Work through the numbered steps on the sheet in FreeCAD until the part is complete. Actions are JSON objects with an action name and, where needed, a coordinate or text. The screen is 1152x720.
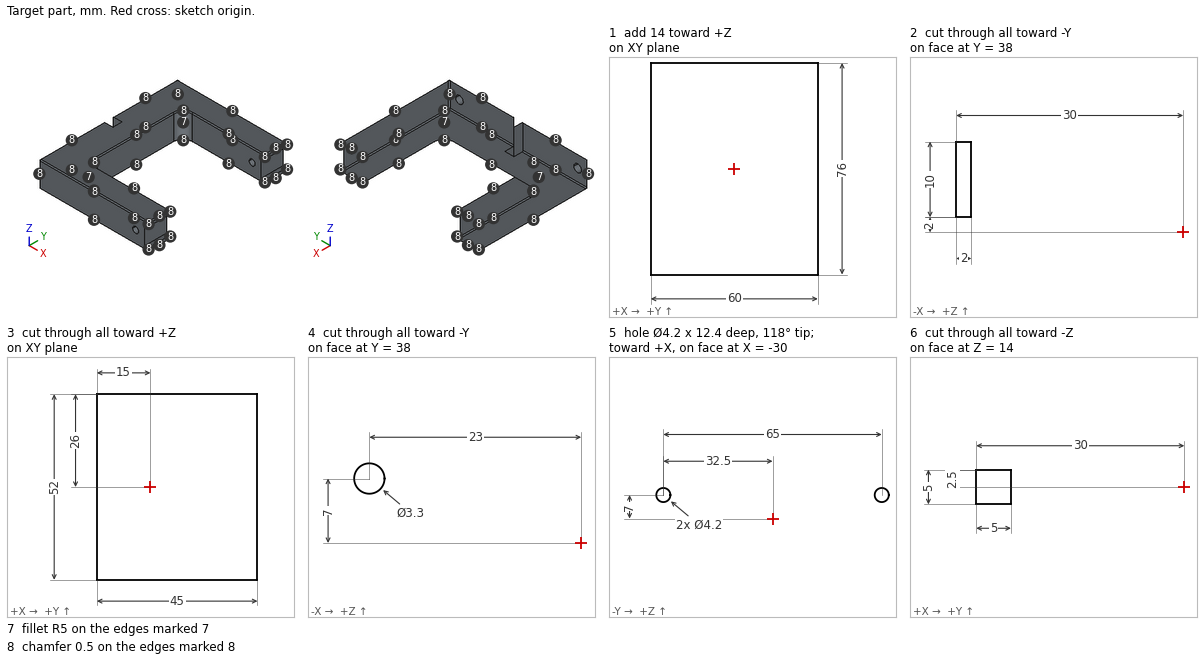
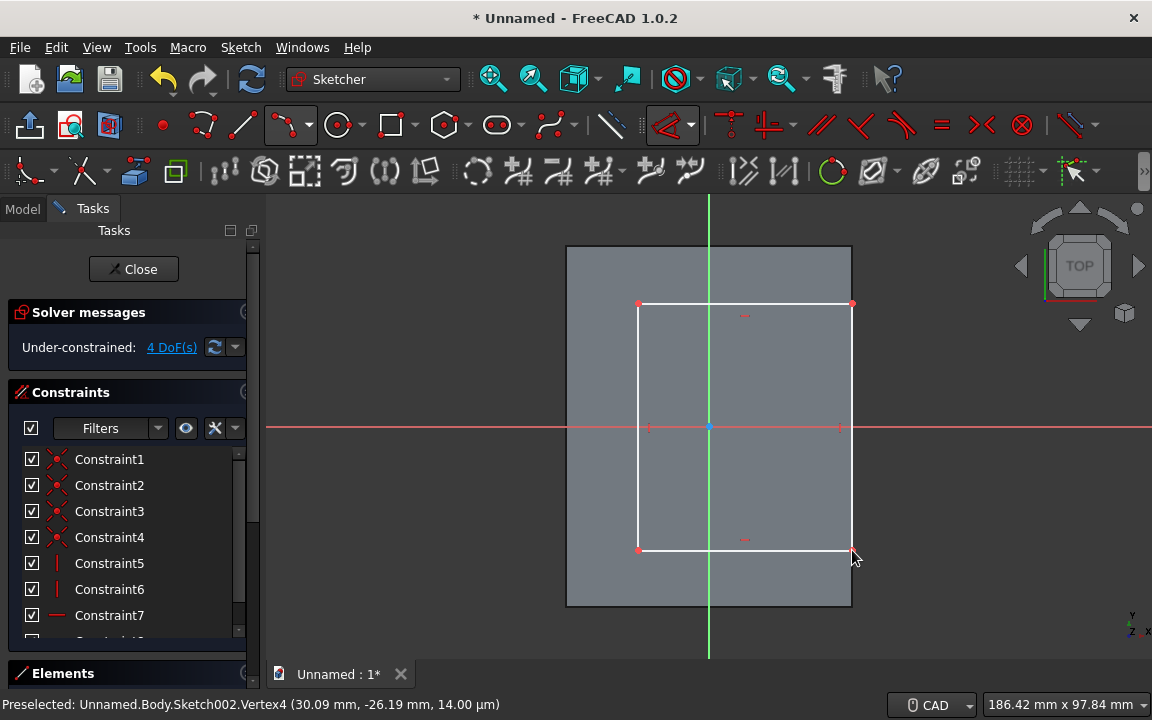
{"action": "left_click", "coordinate": [638, 378]}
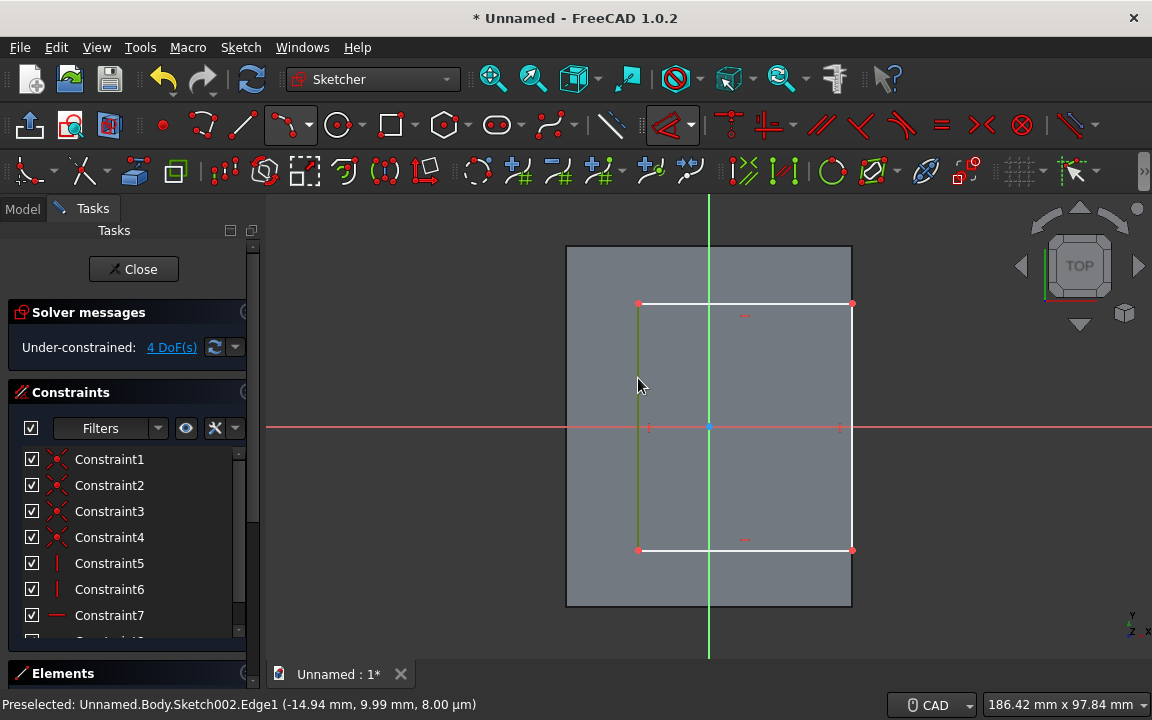
{"action": "key", "text": "i"}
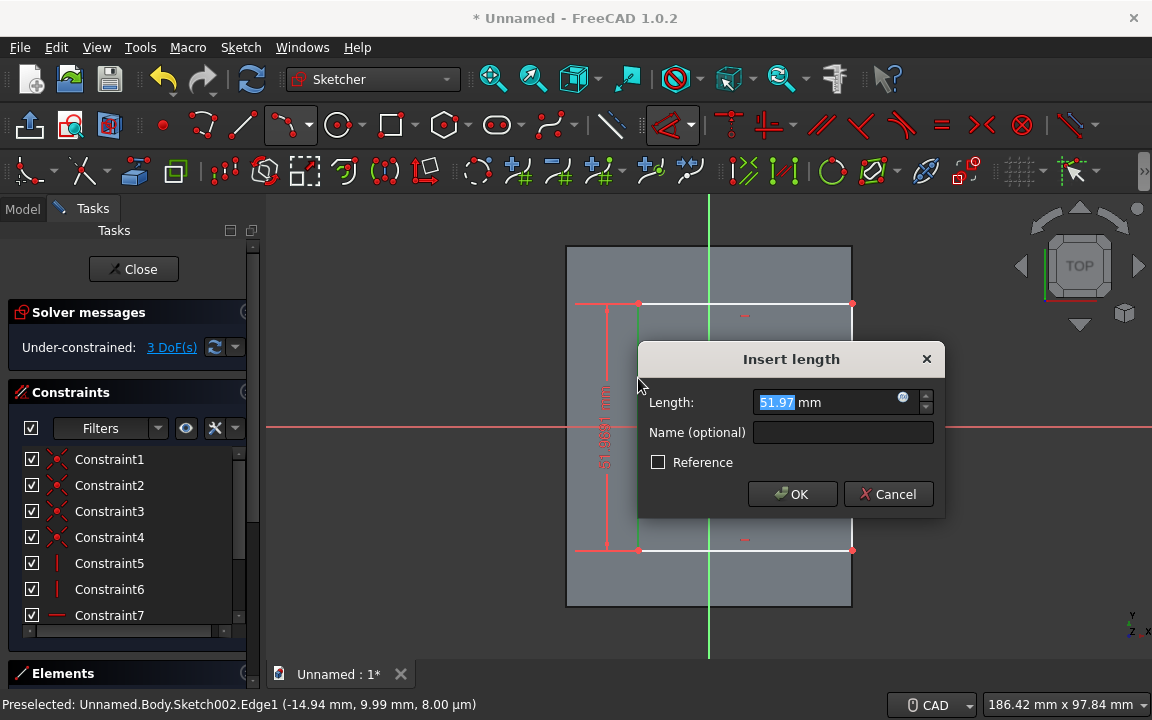
{"action": "type", "text": "52"}
{"action": "key", "text": "Return"}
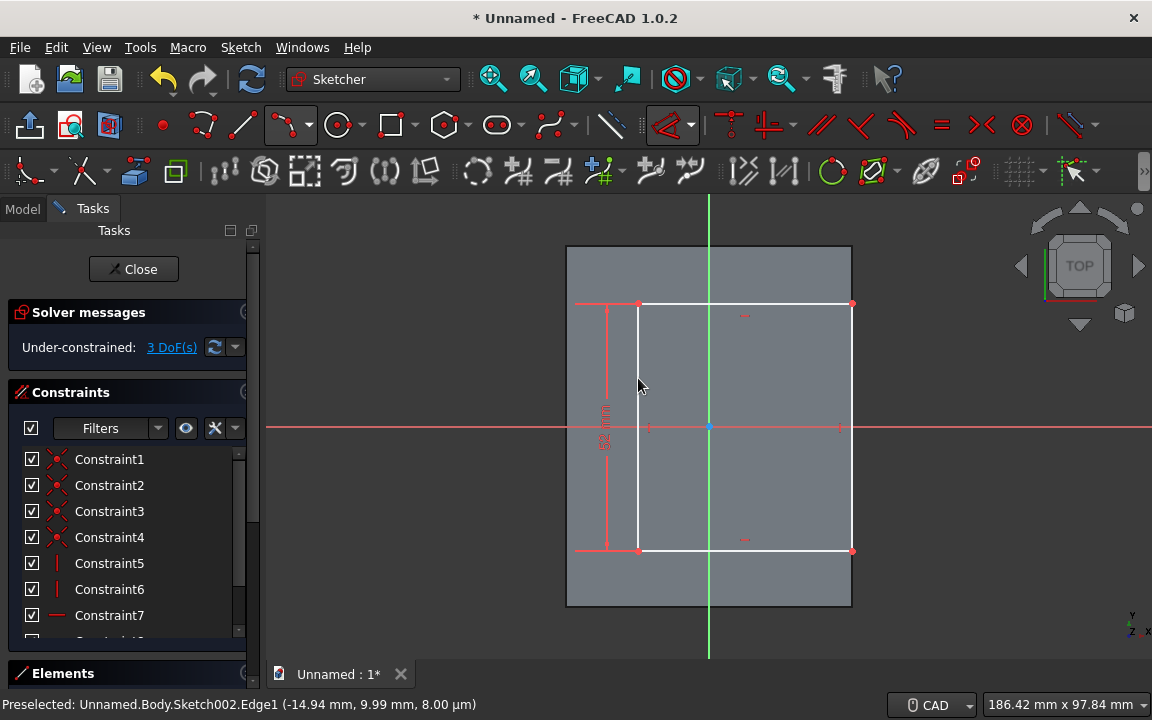
{"action": "left_click", "coordinate": [788, 551]}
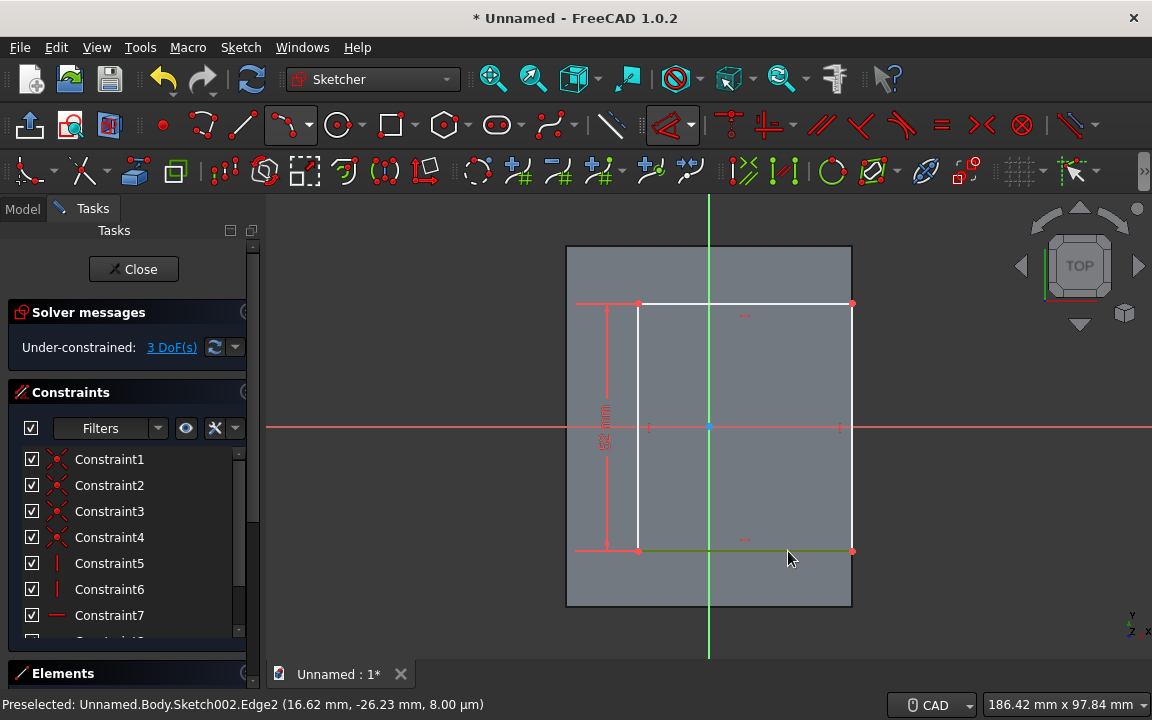
{"action": "key", "text": "l"}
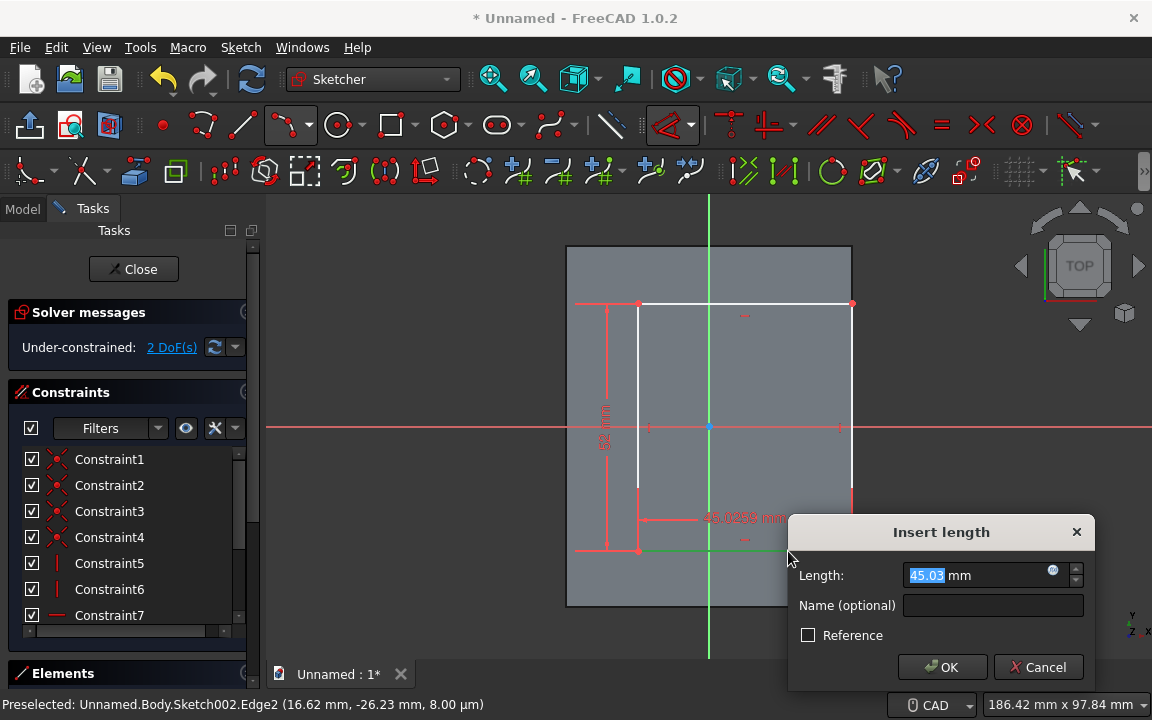
{"action": "type", "text": "45"}
{"action": "key", "text": "Return"}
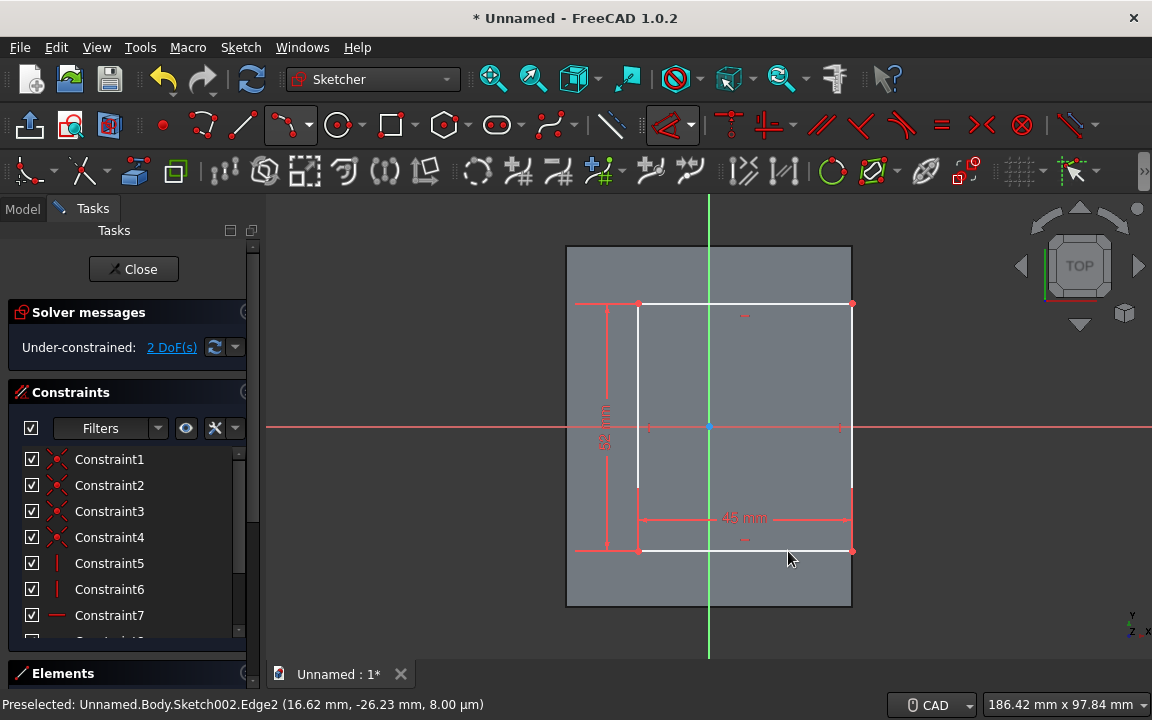
{"action": "left_click", "coordinate": [638, 304]}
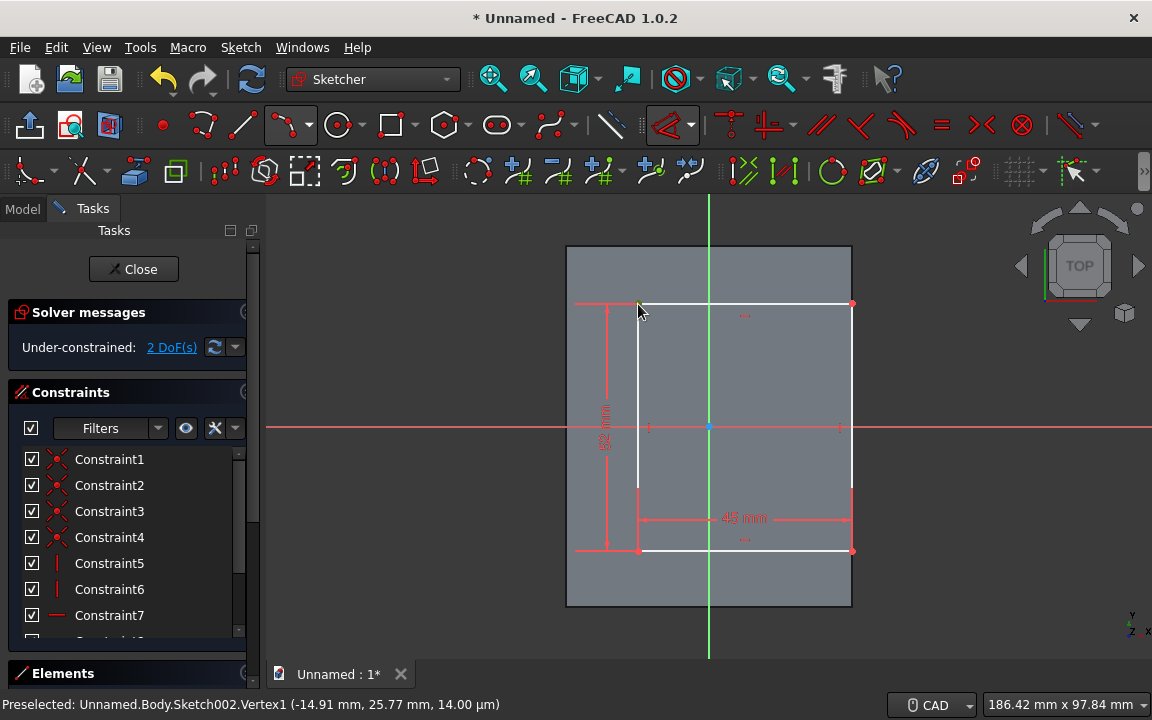
{"action": "key", "text": "l"}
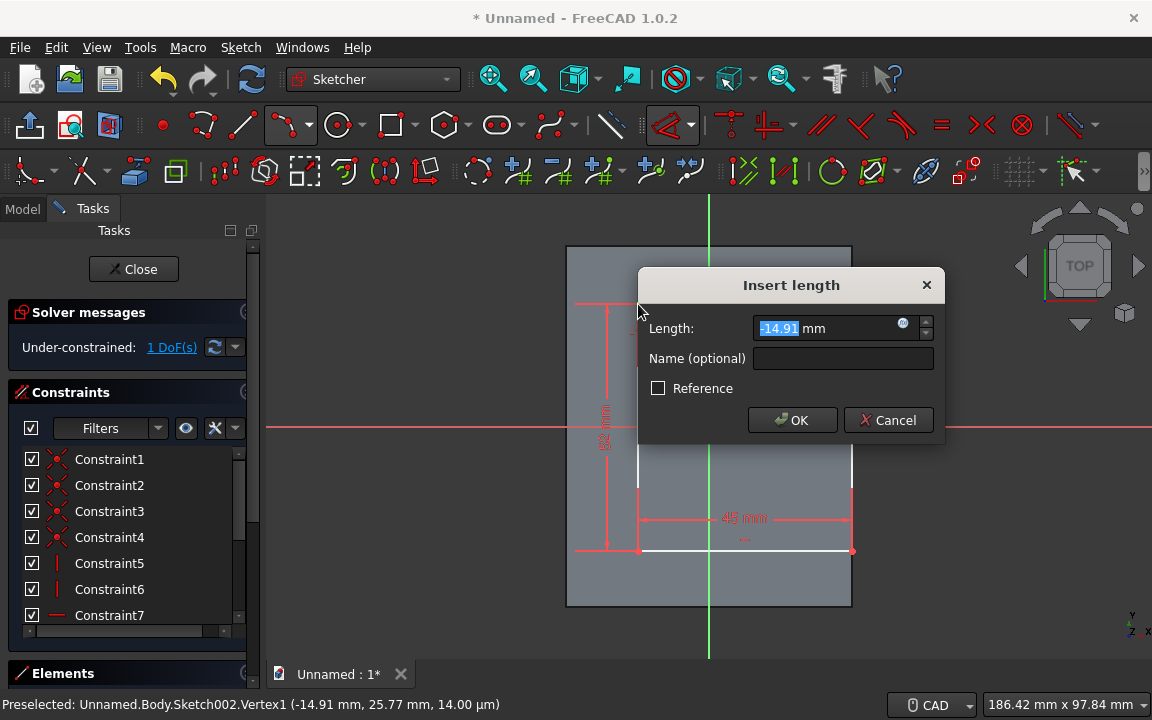
{"action": "type", "text": "-15"}
{"action": "key", "text": "Return"}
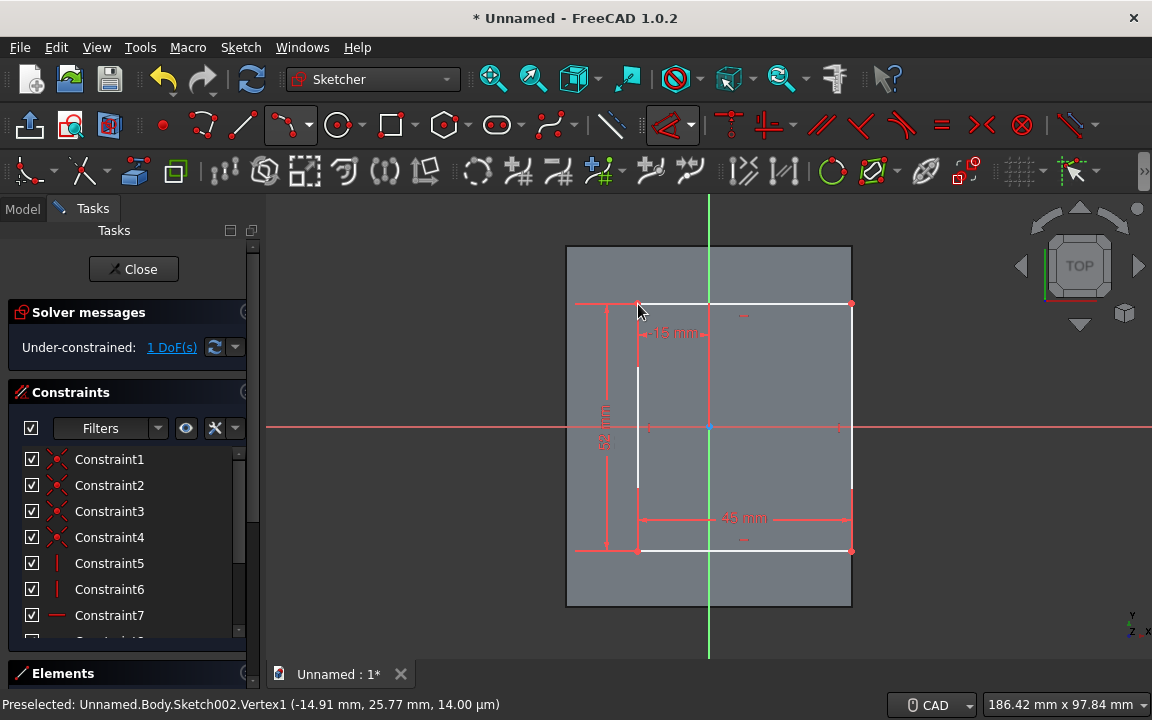
{"action": "left_click", "coordinate": [638, 304]}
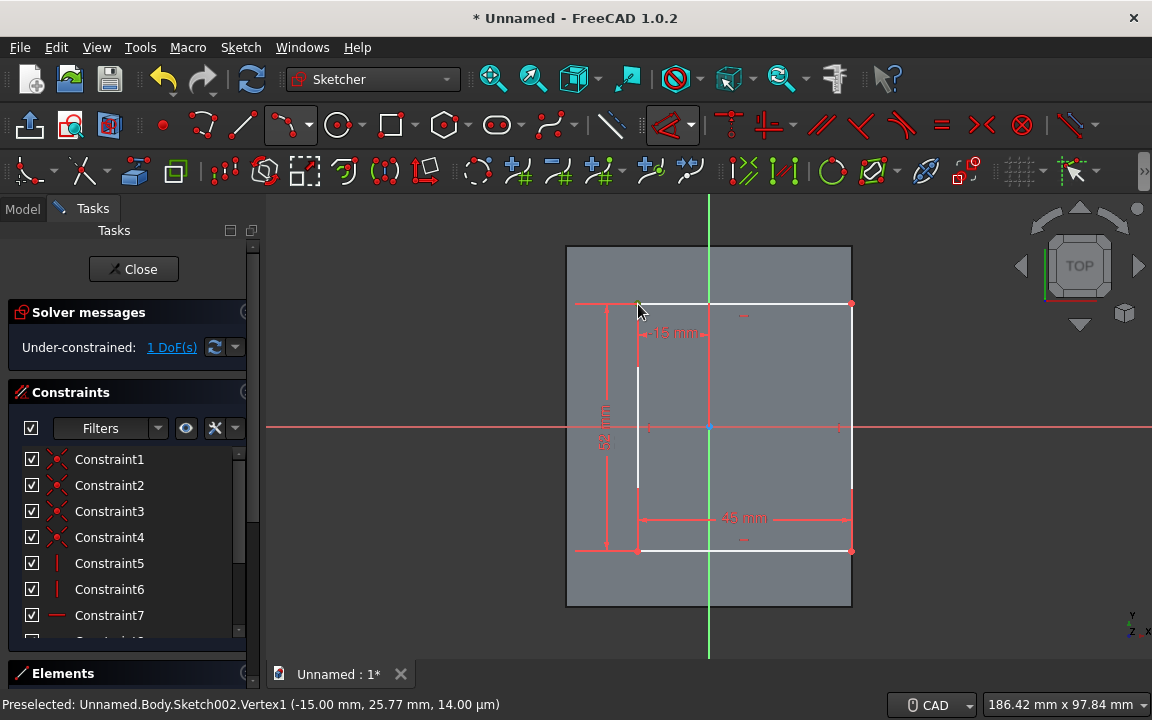
{"action": "key", "text": "i"}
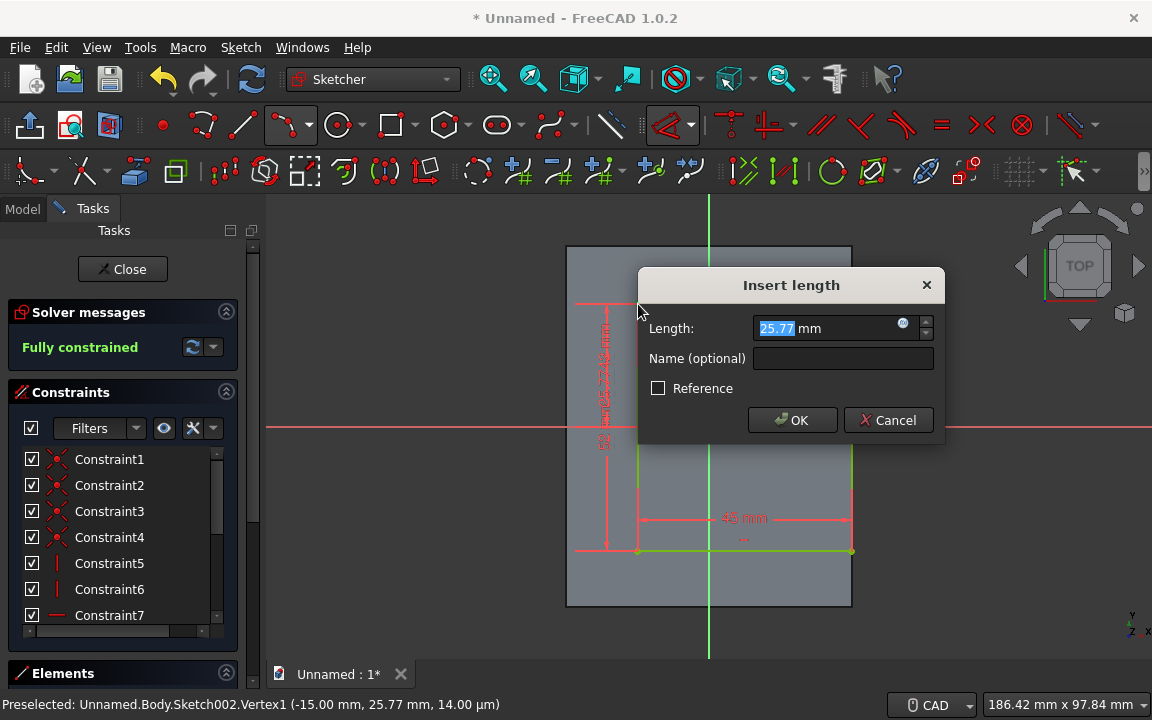
{"action": "type", "text": "26"}
{"action": "key", "text": "Return"}